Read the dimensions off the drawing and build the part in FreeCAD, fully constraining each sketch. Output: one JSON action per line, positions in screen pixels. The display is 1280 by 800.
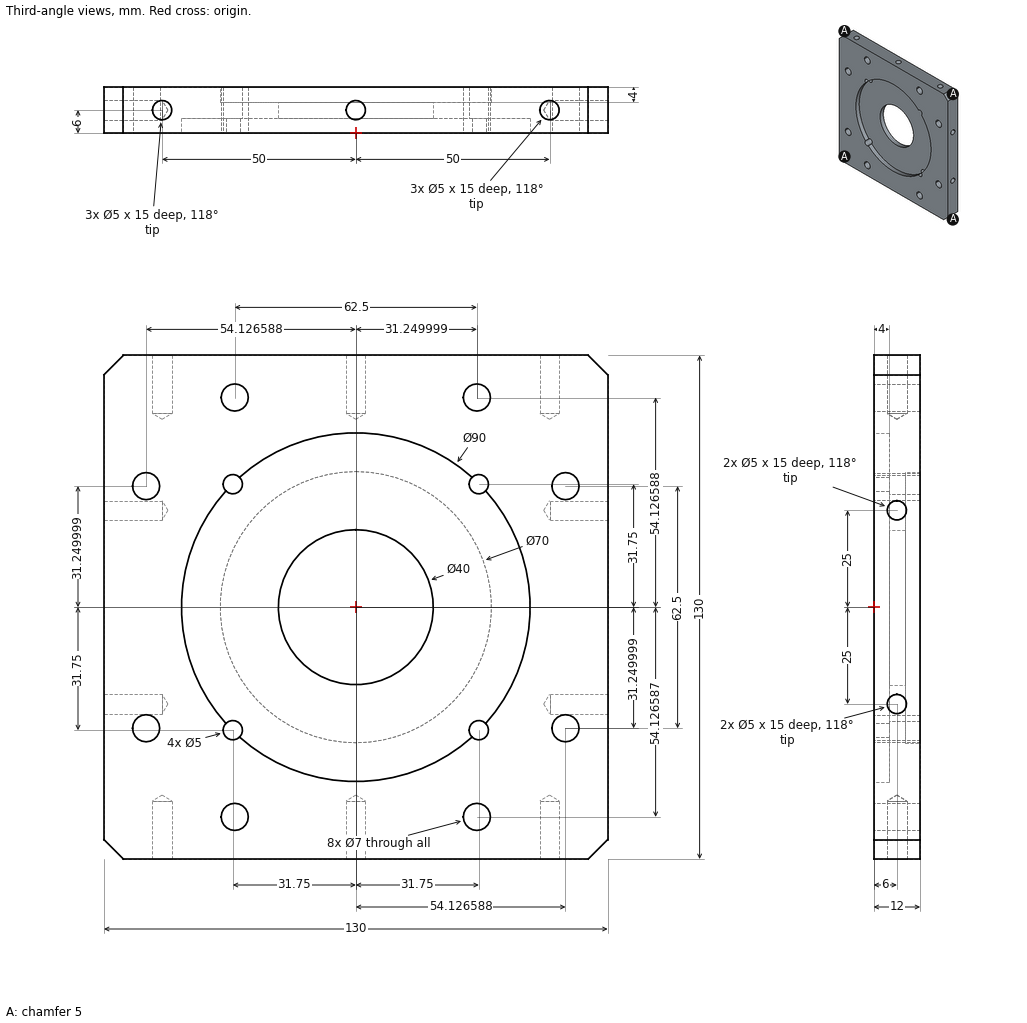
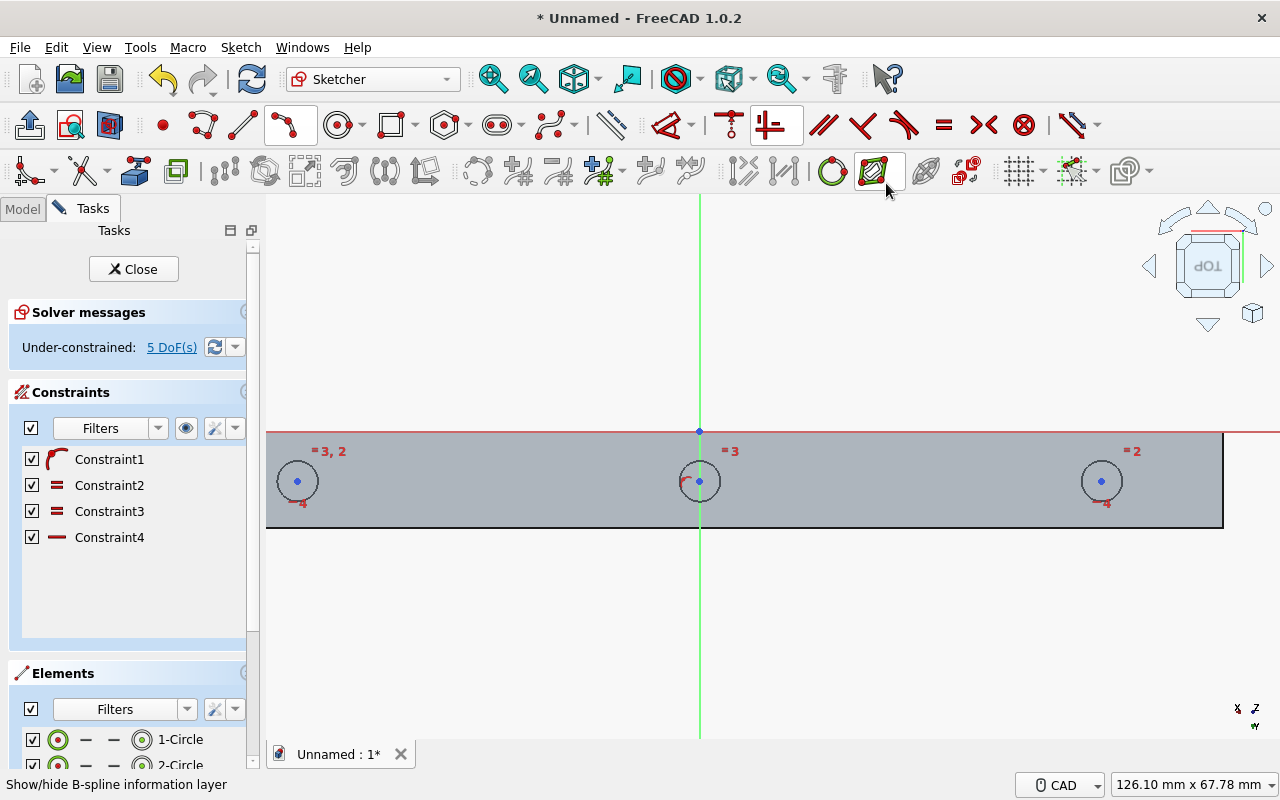
{"action": "left_click", "coordinate": [1102, 481]}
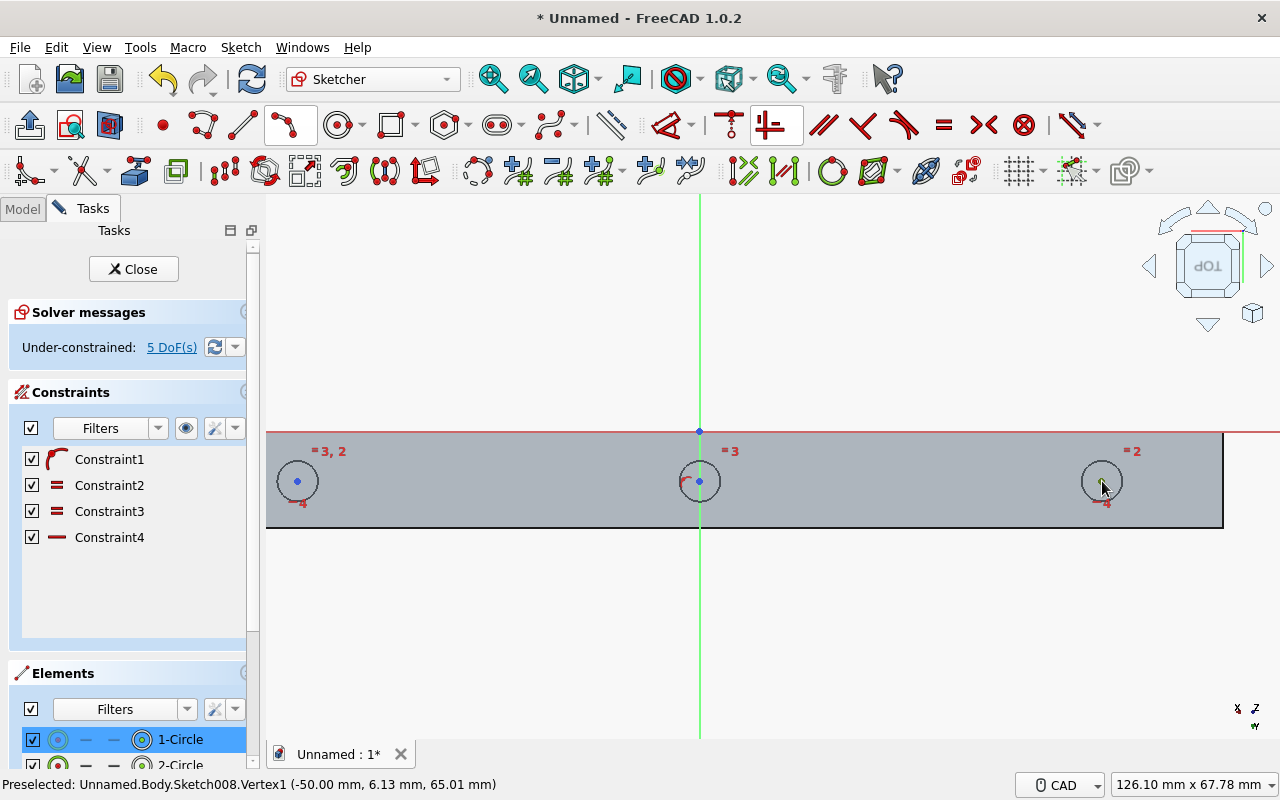
{"action": "left_click", "coordinate": [700, 481]}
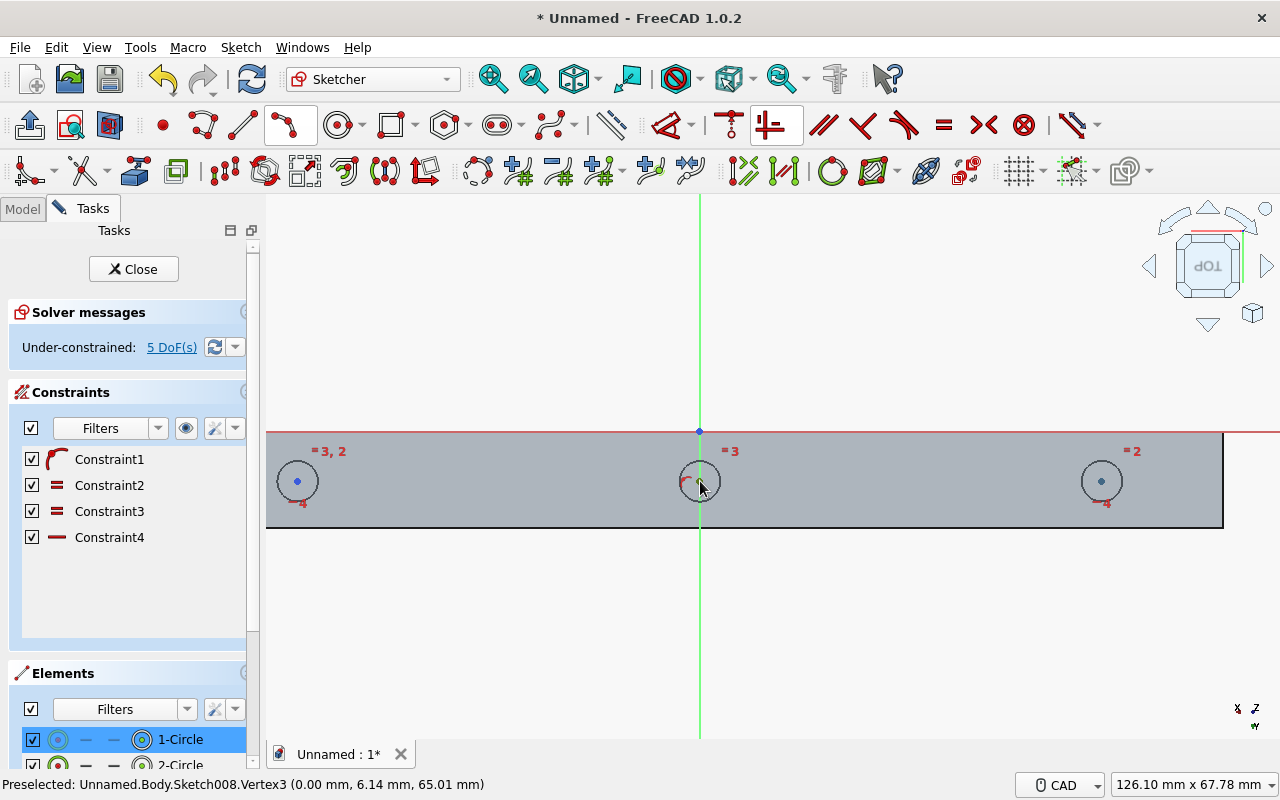
{"action": "key", "text": "h"}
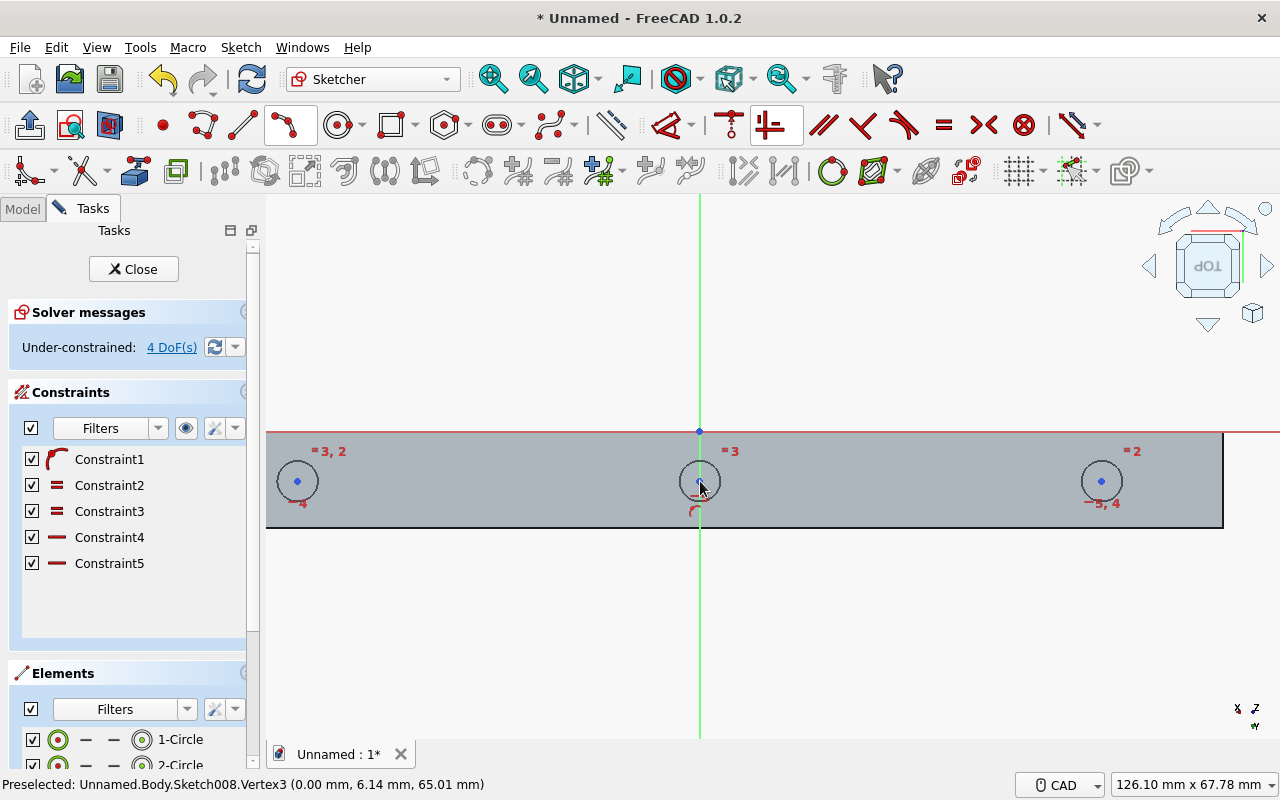
{"action": "left_click", "coordinate": [666, 126]}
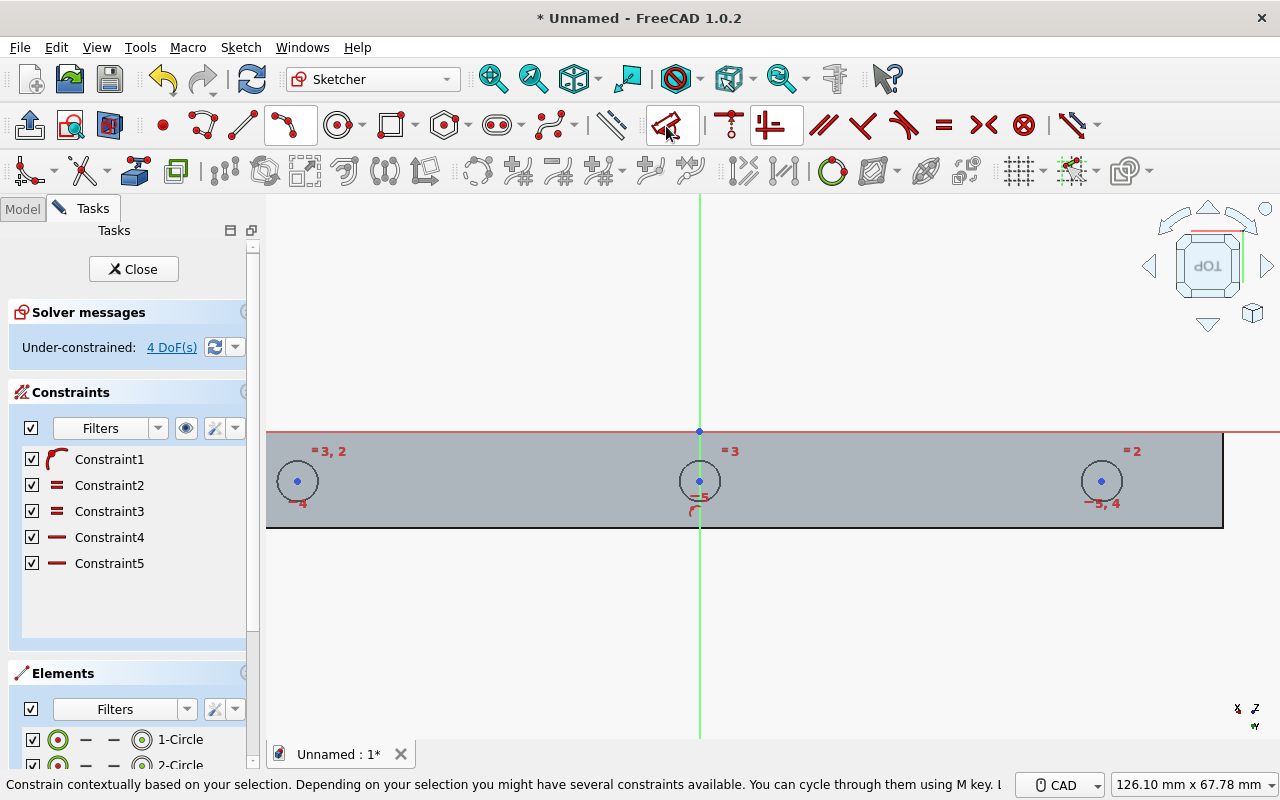
{"action": "left_click", "coordinate": [1088, 467]}
{"action": "left_click", "coordinate": [1052, 466]}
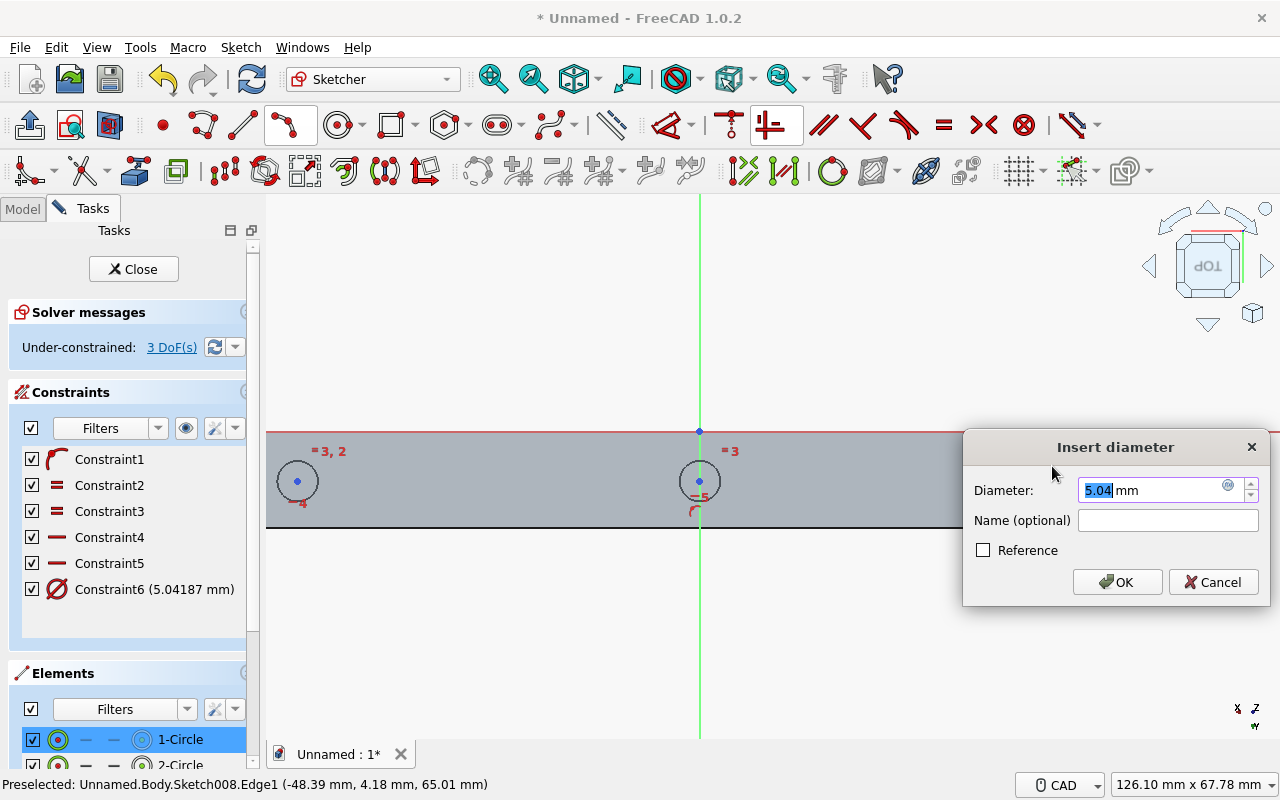
{"action": "type", "text": "5"}
{"action": "key", "text": "Return"}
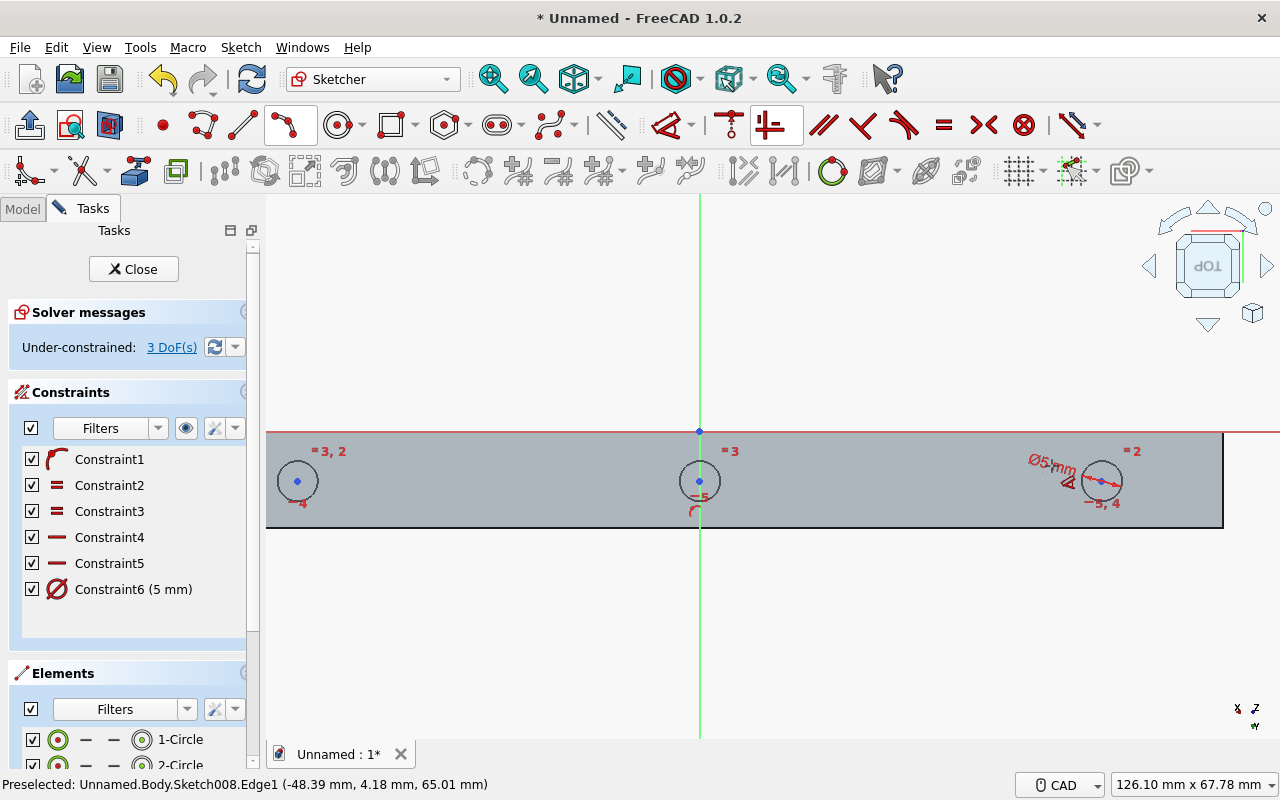
{"action": "left_click", "coordinate": [1102, 481]}
{"action": "left_click", "coordinate": [666, 457]}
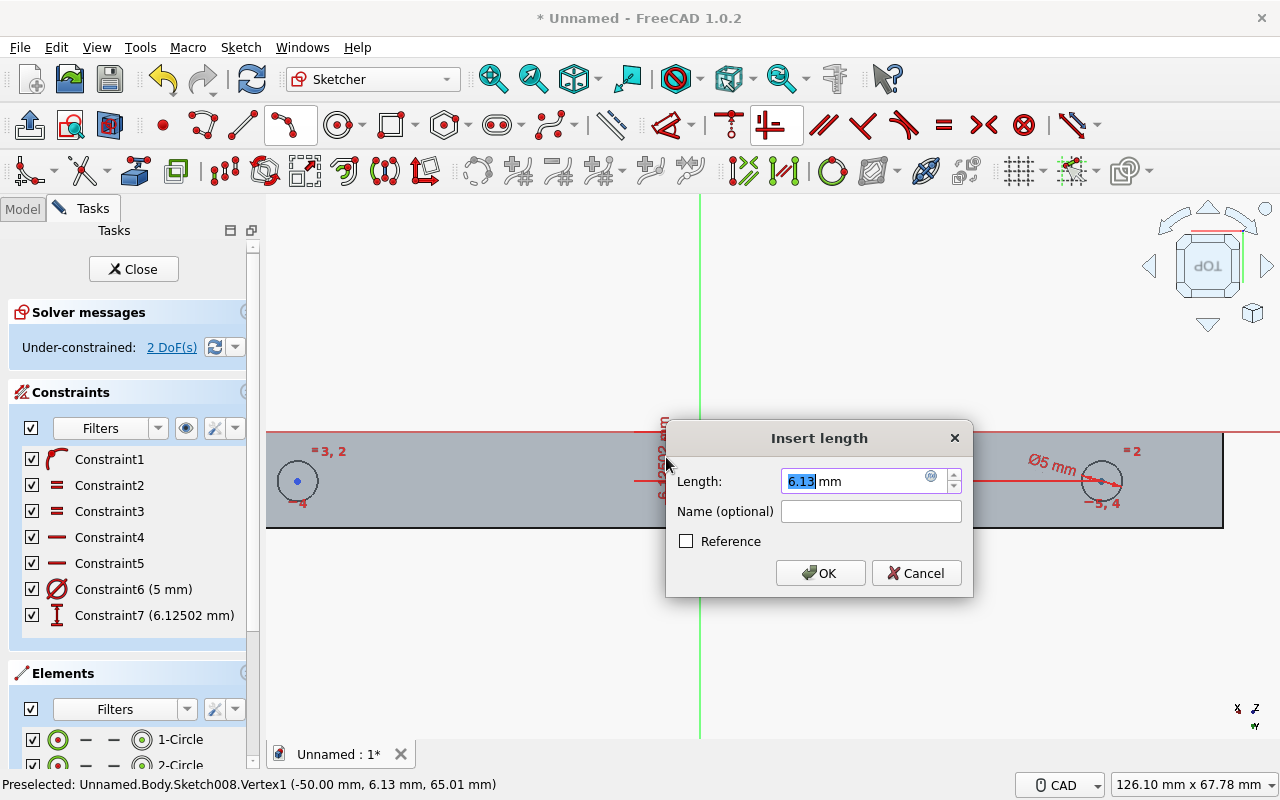
{"action": "type", "text": "6"}
{"action": "key", "text": "Return"}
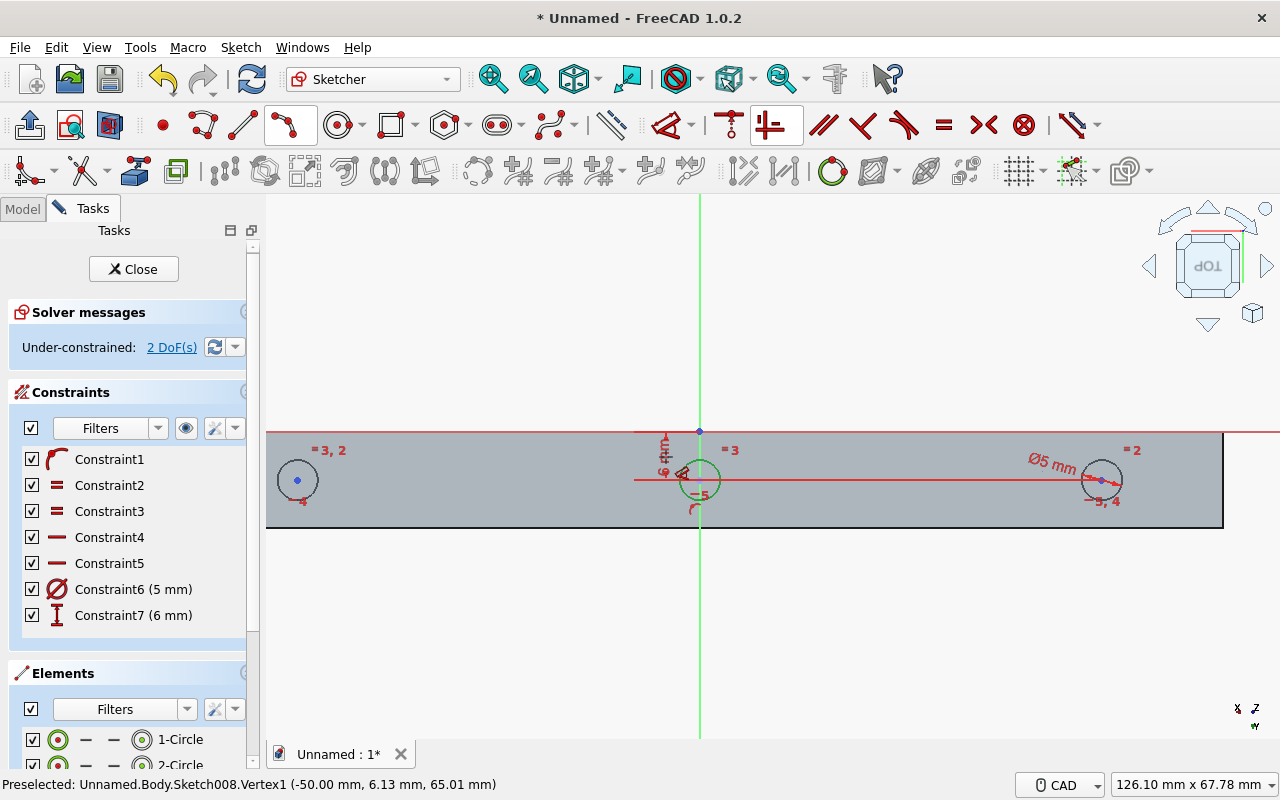
{"action": "left_click", "coordinate": [1102, 480]}
{"action": "left_click", "coordinate": [901, 398]}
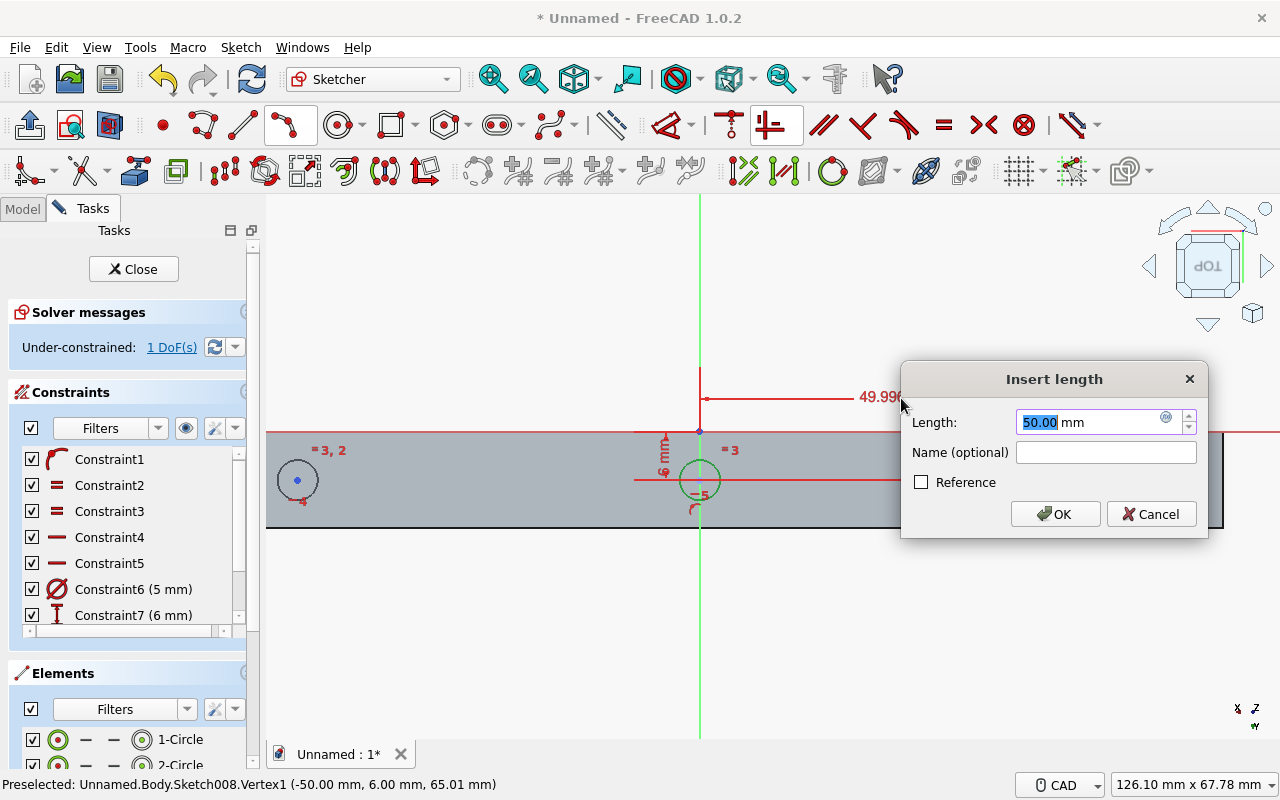
{"action": "type", "text": "50"}
{"action": "key", "text": "Return"}